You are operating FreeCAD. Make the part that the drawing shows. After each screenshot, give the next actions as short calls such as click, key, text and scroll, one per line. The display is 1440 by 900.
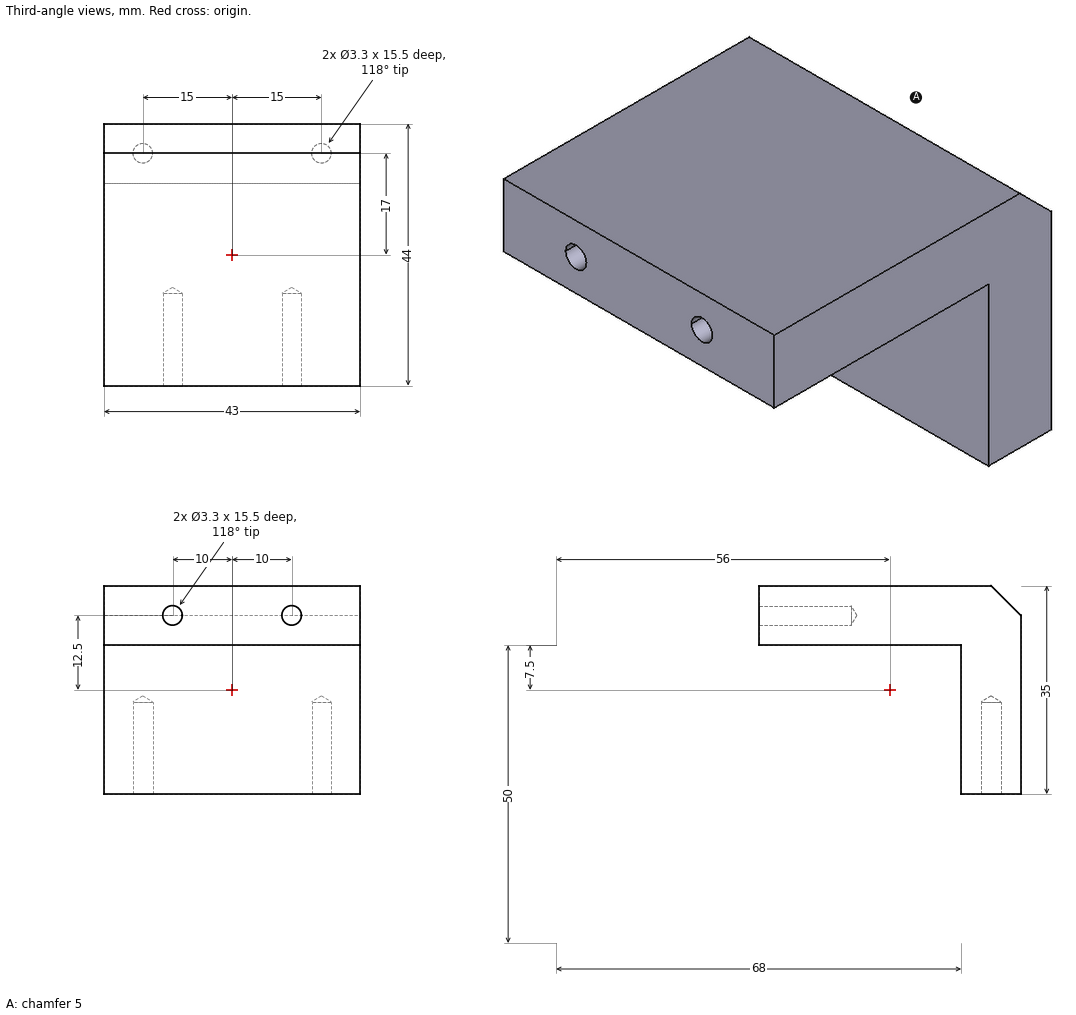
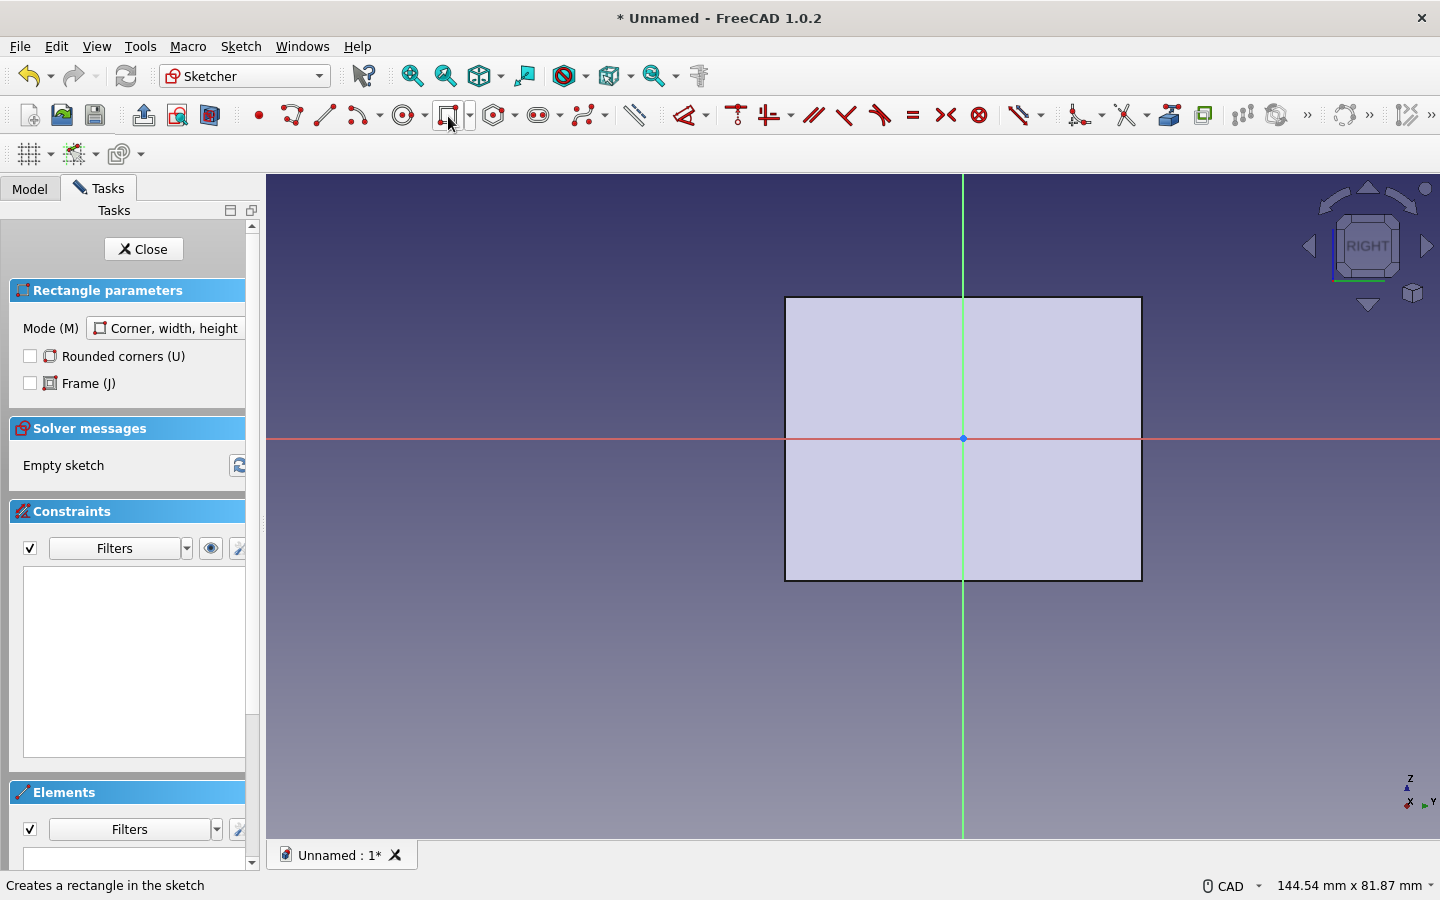
click(508, 378)
click(1061, 784)
key(Escape)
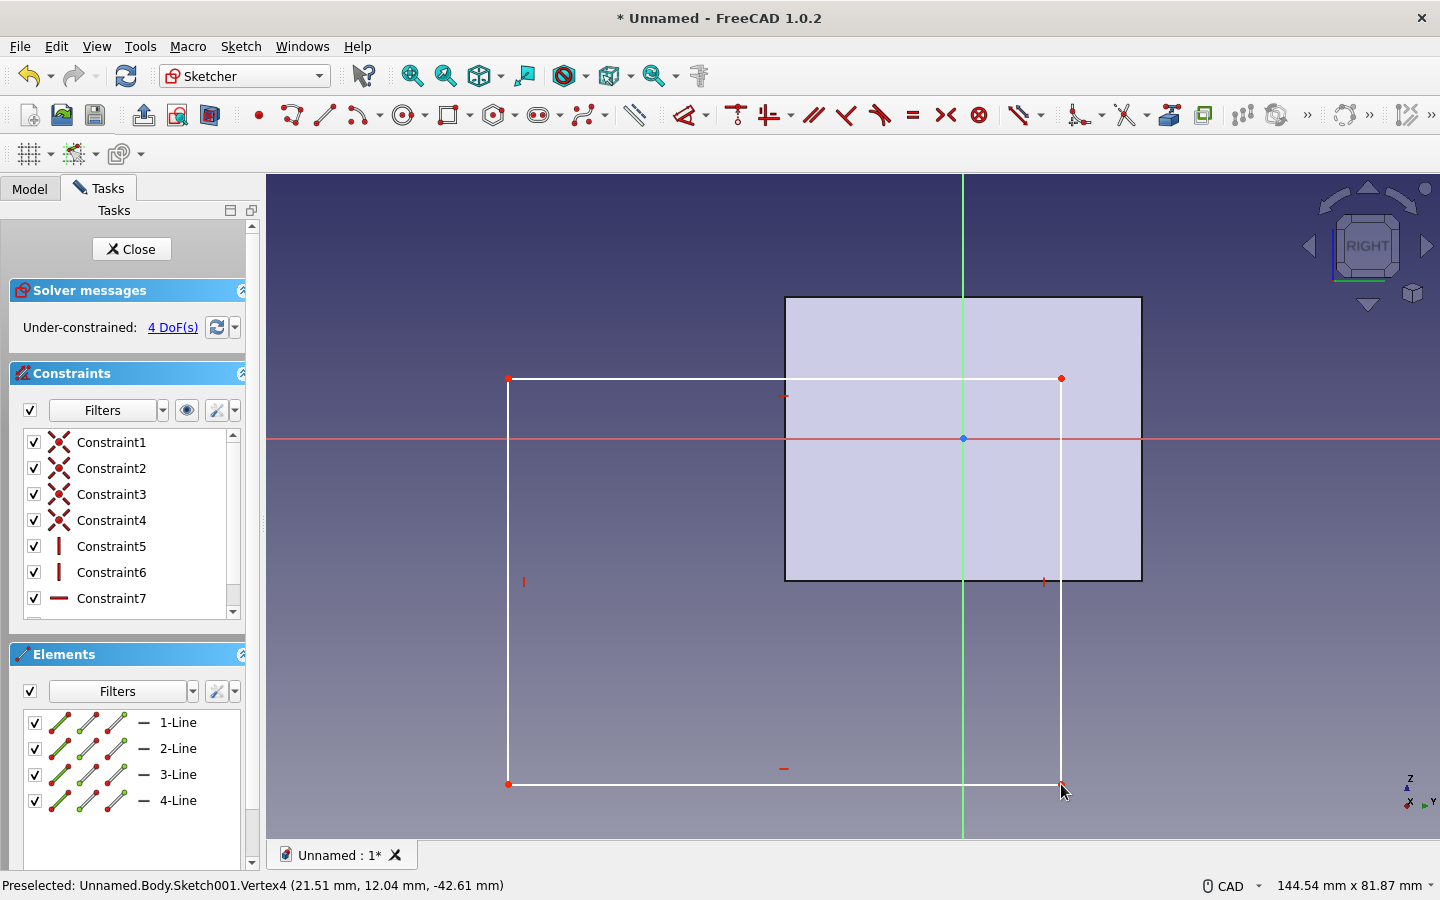
click(684, 116)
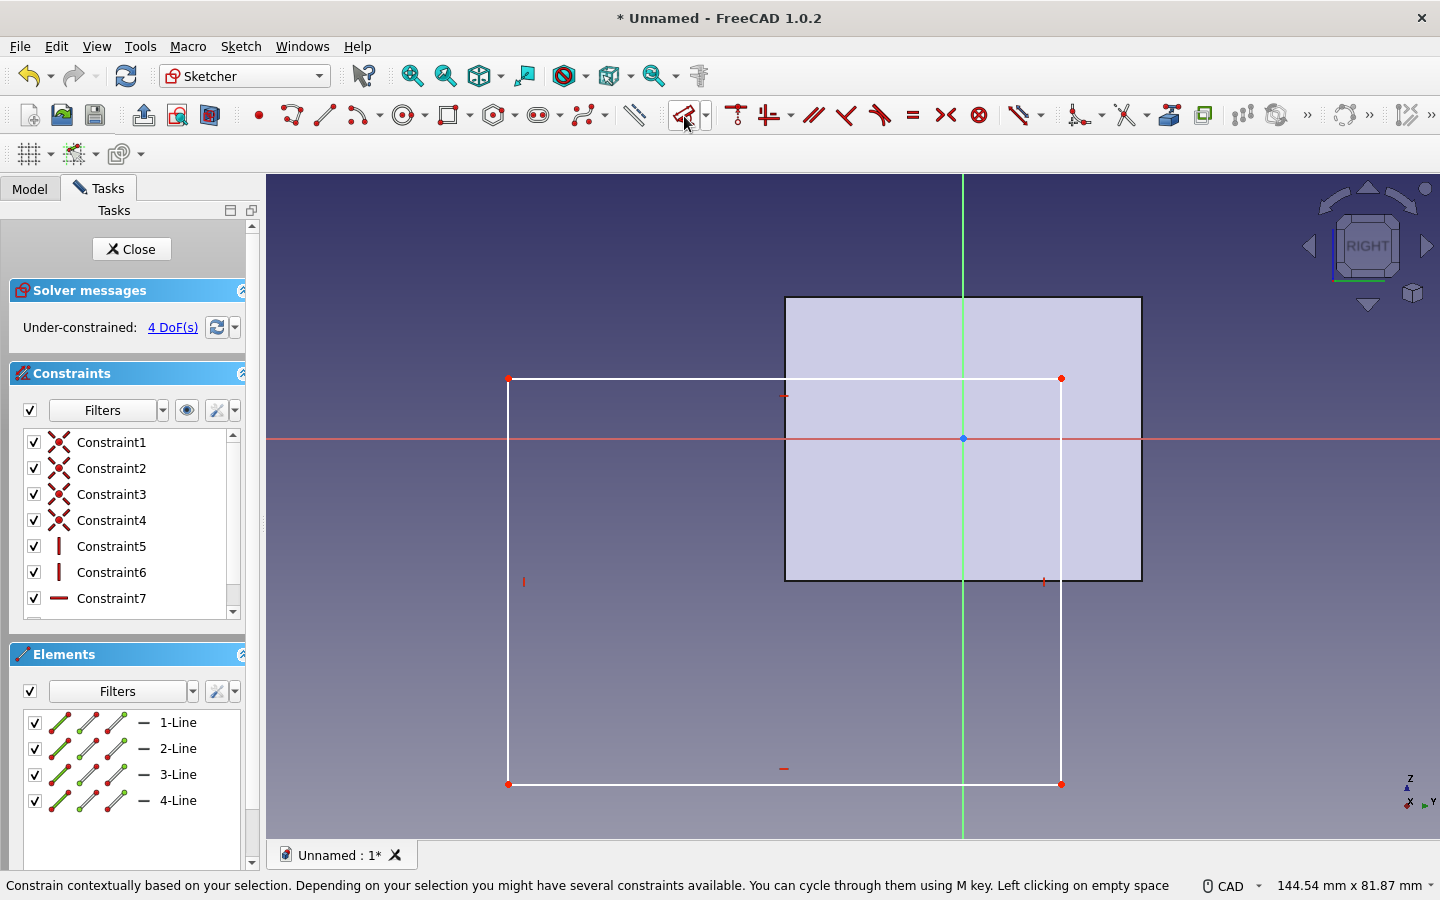
click(508, 501)
click(474, 582)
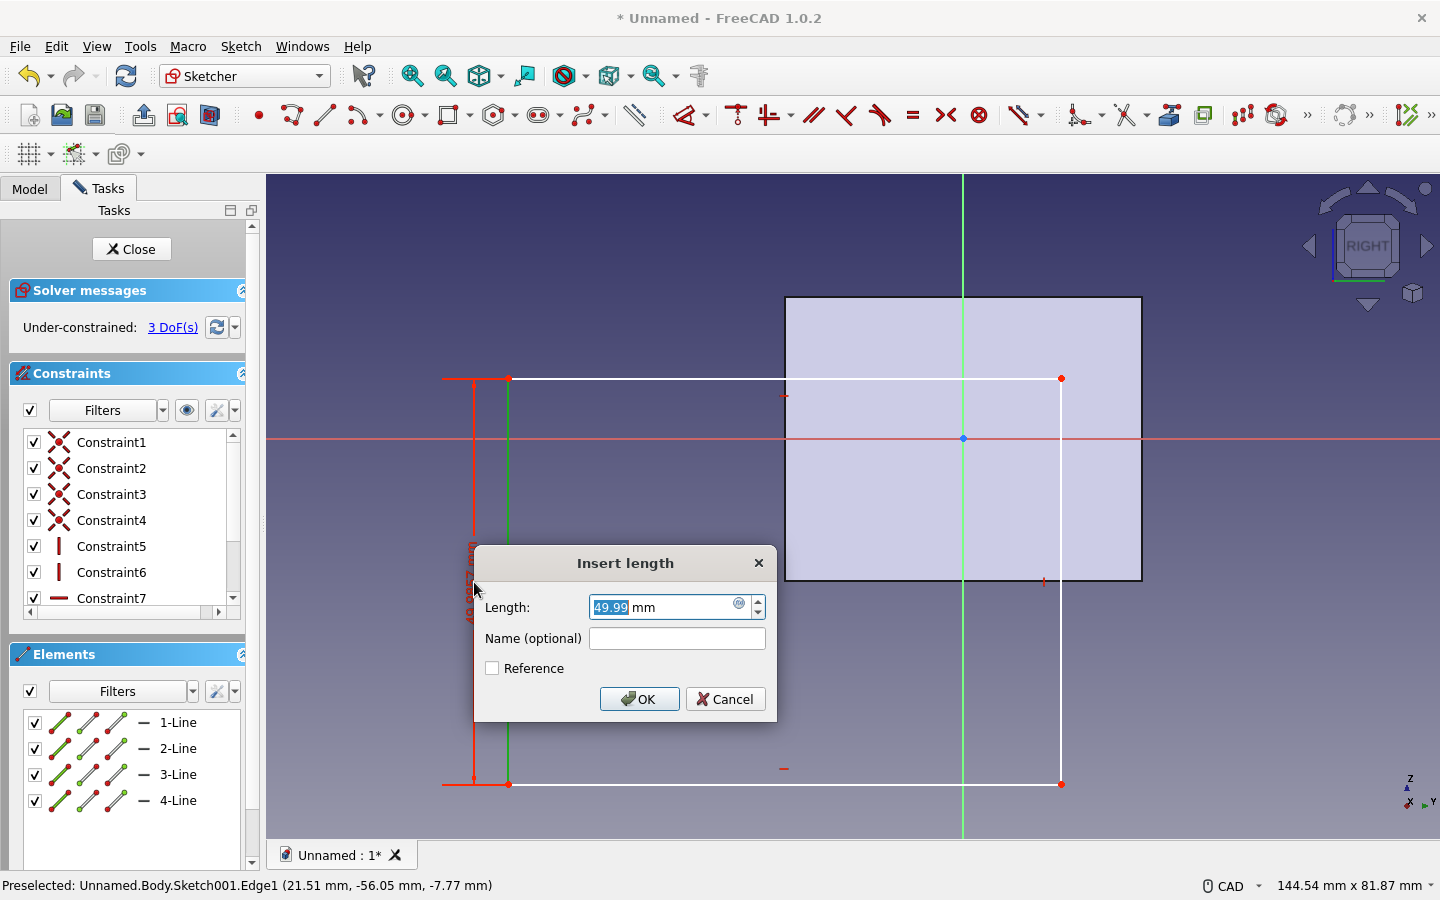
text(50)
key(Return)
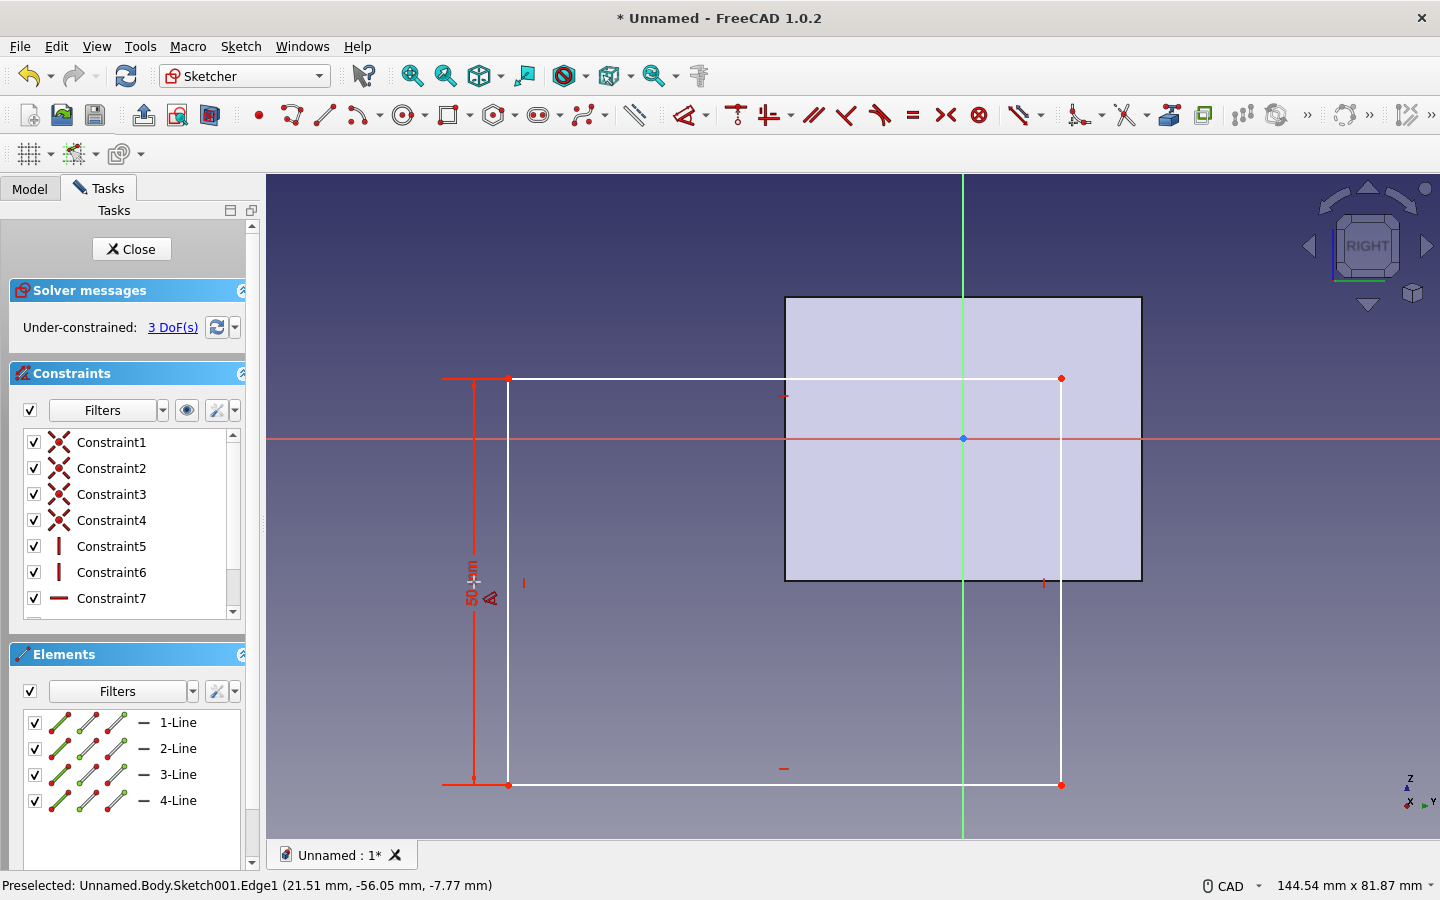
click(674, 785)
click(784, 751)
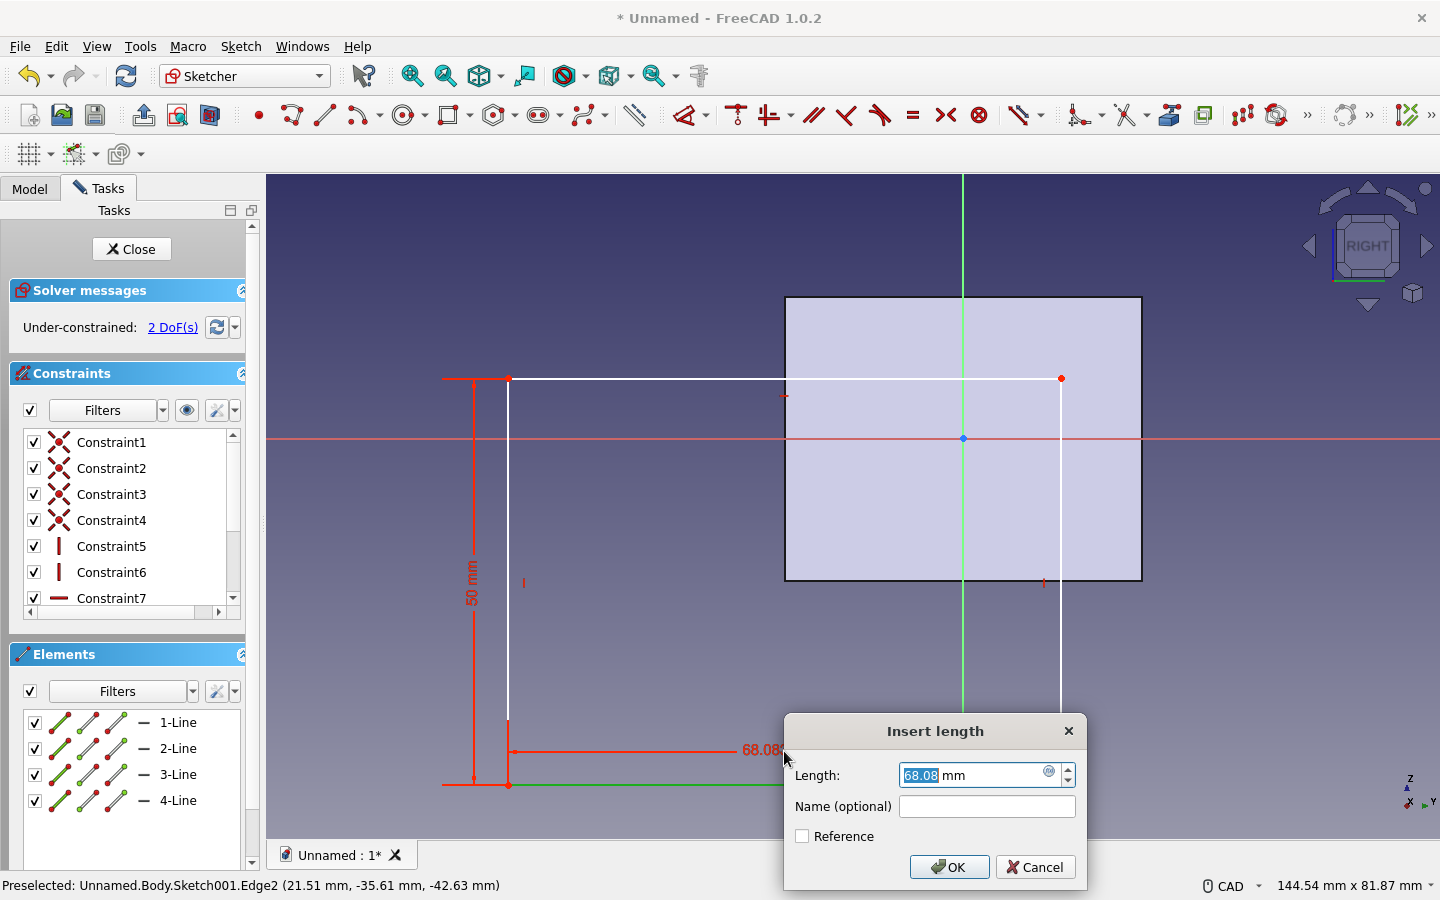
text(68)
key(Return)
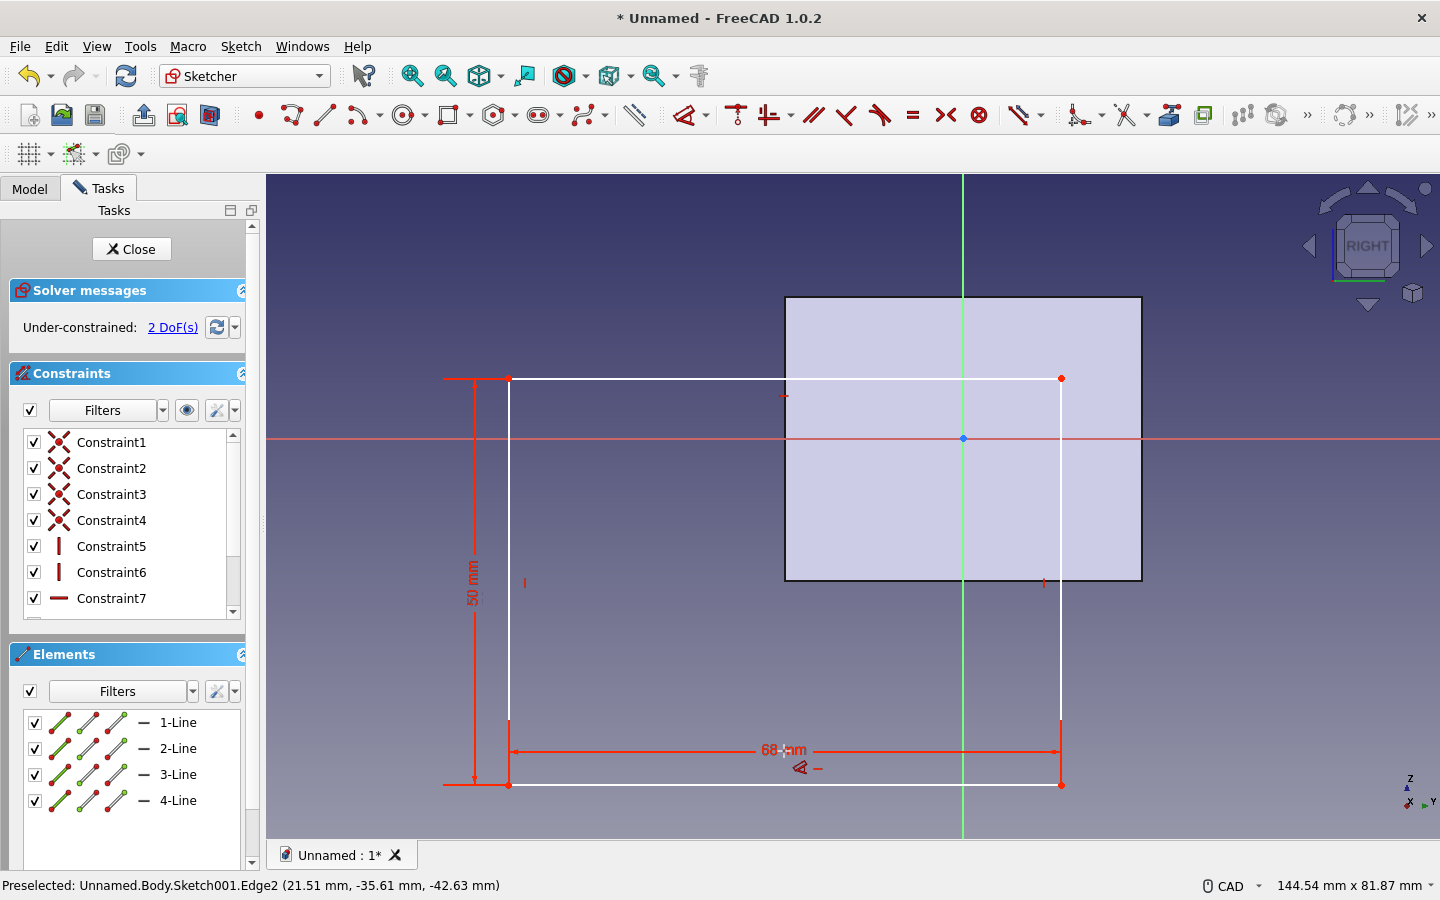
click(509, 379)
click(736, 345)